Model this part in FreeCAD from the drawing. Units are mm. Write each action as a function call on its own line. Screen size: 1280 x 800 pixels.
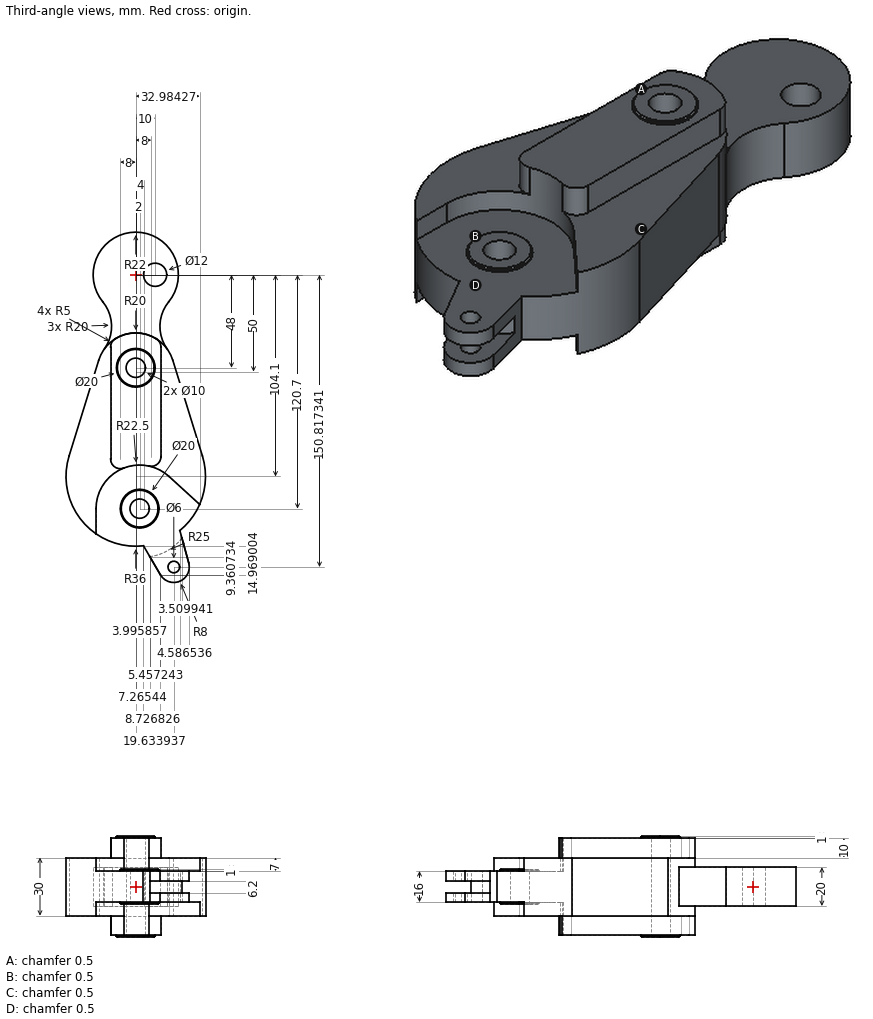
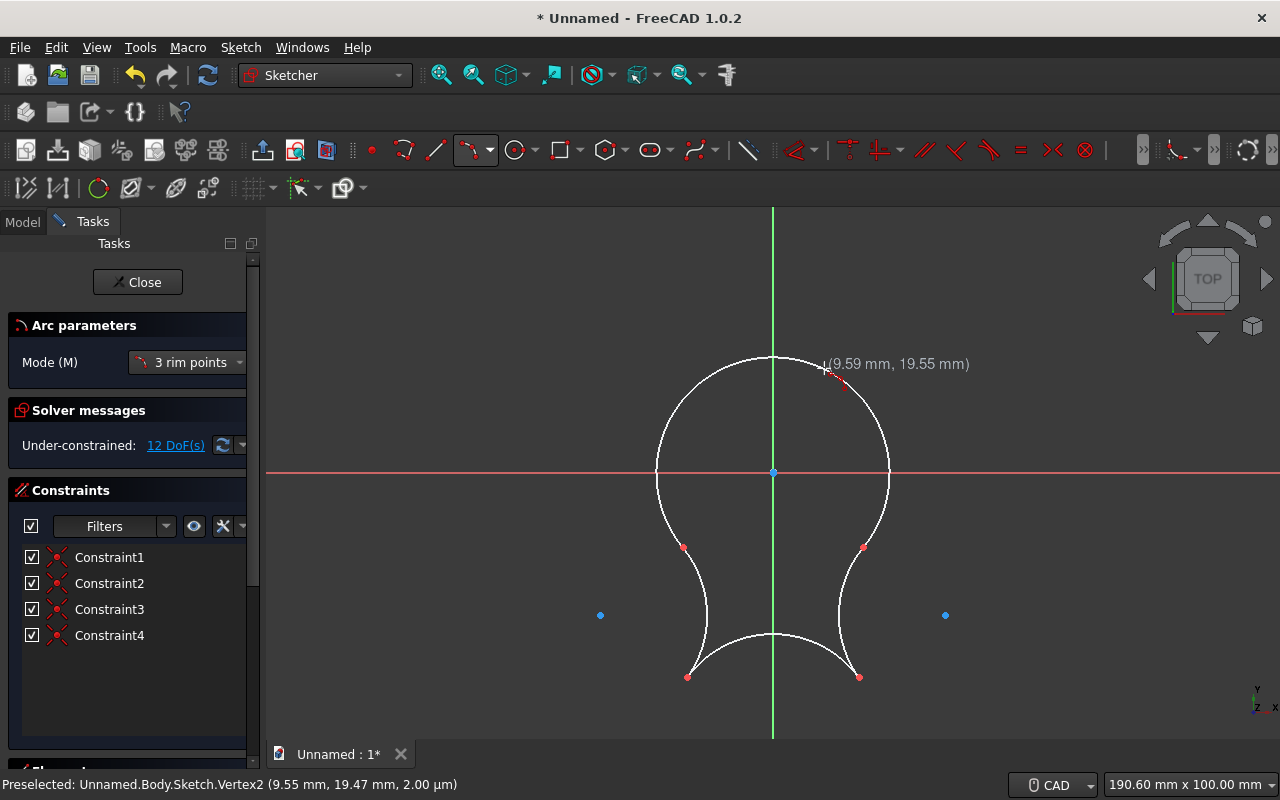
click(516, 150)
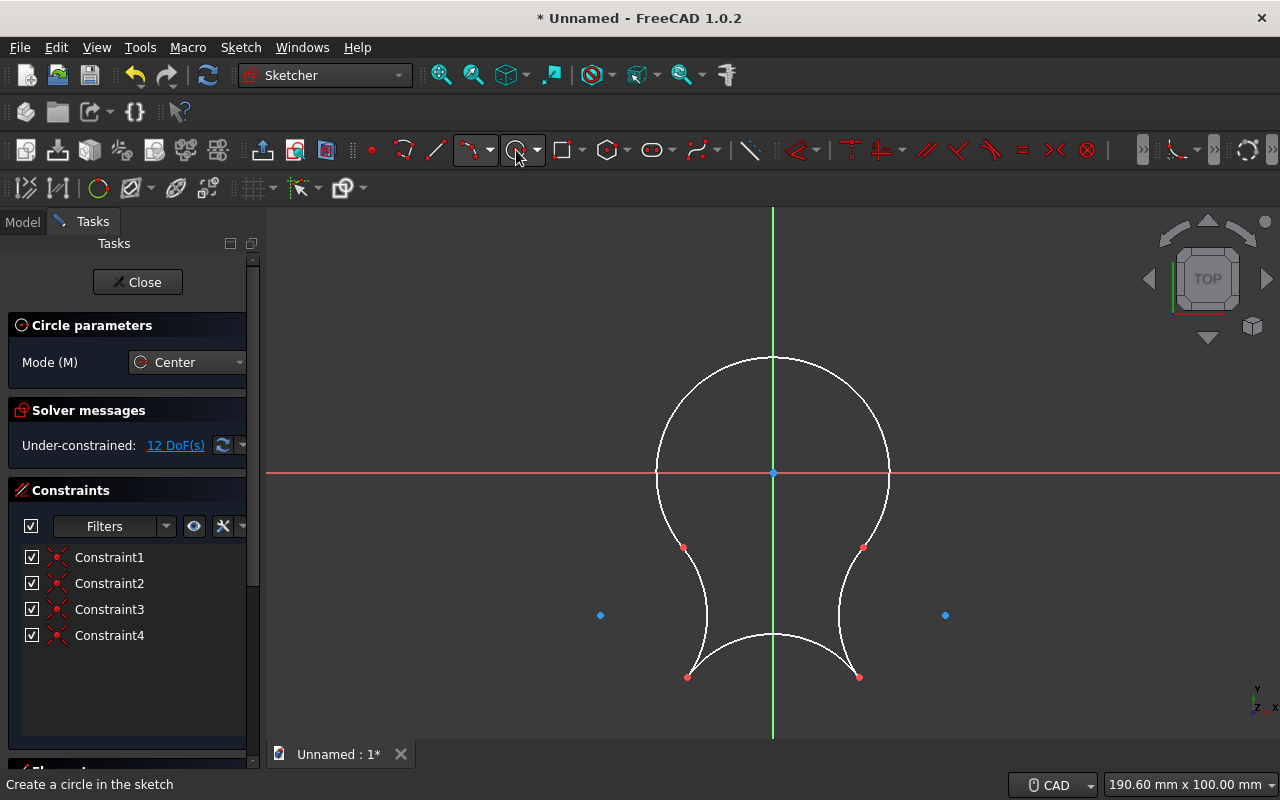
click(826, 473)
click(849, 450)
key(Escape)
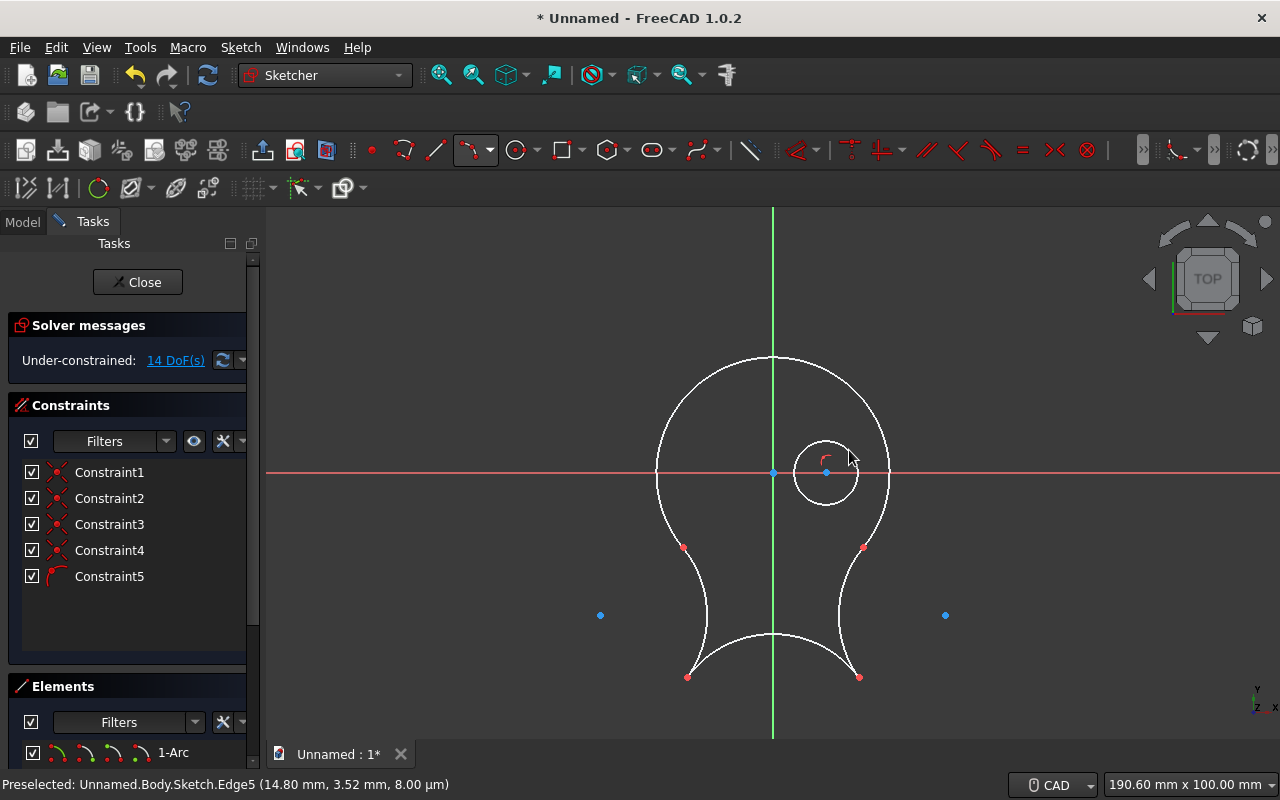
click(704, 640)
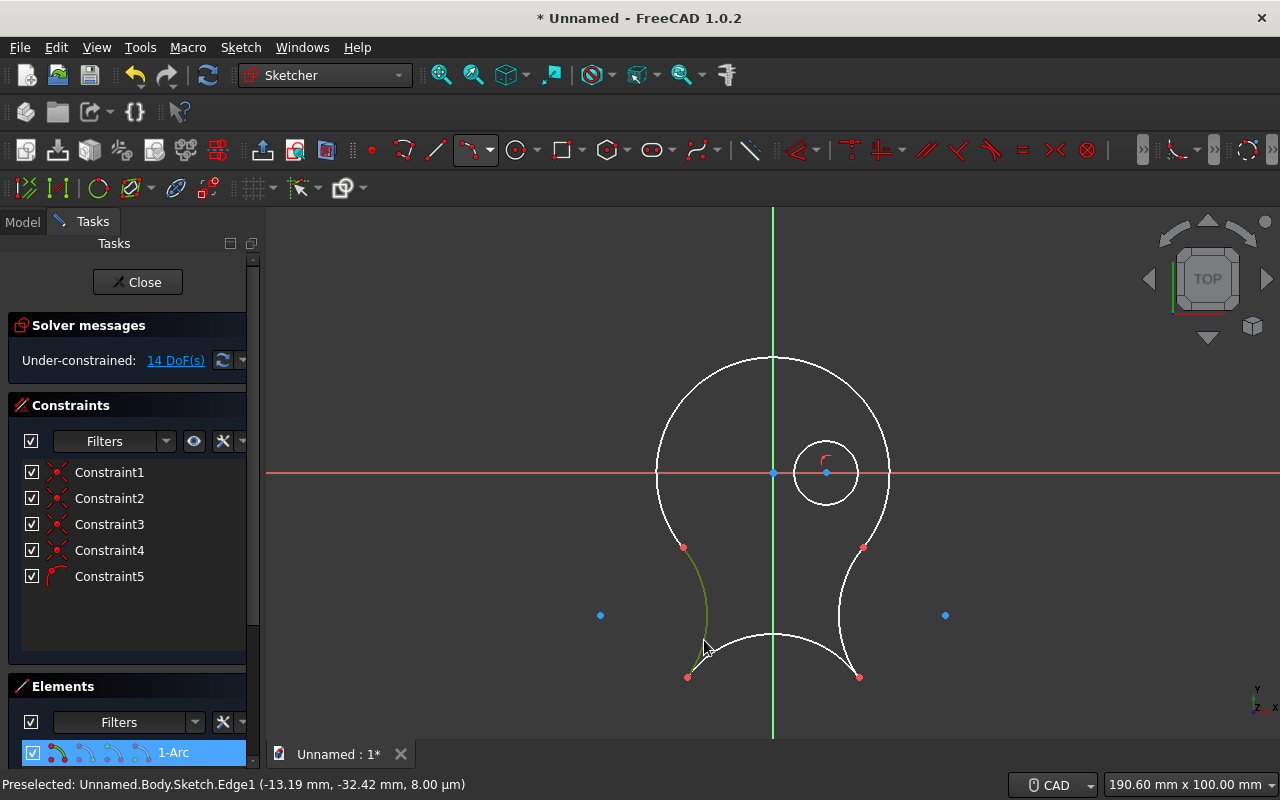
click(812, 642)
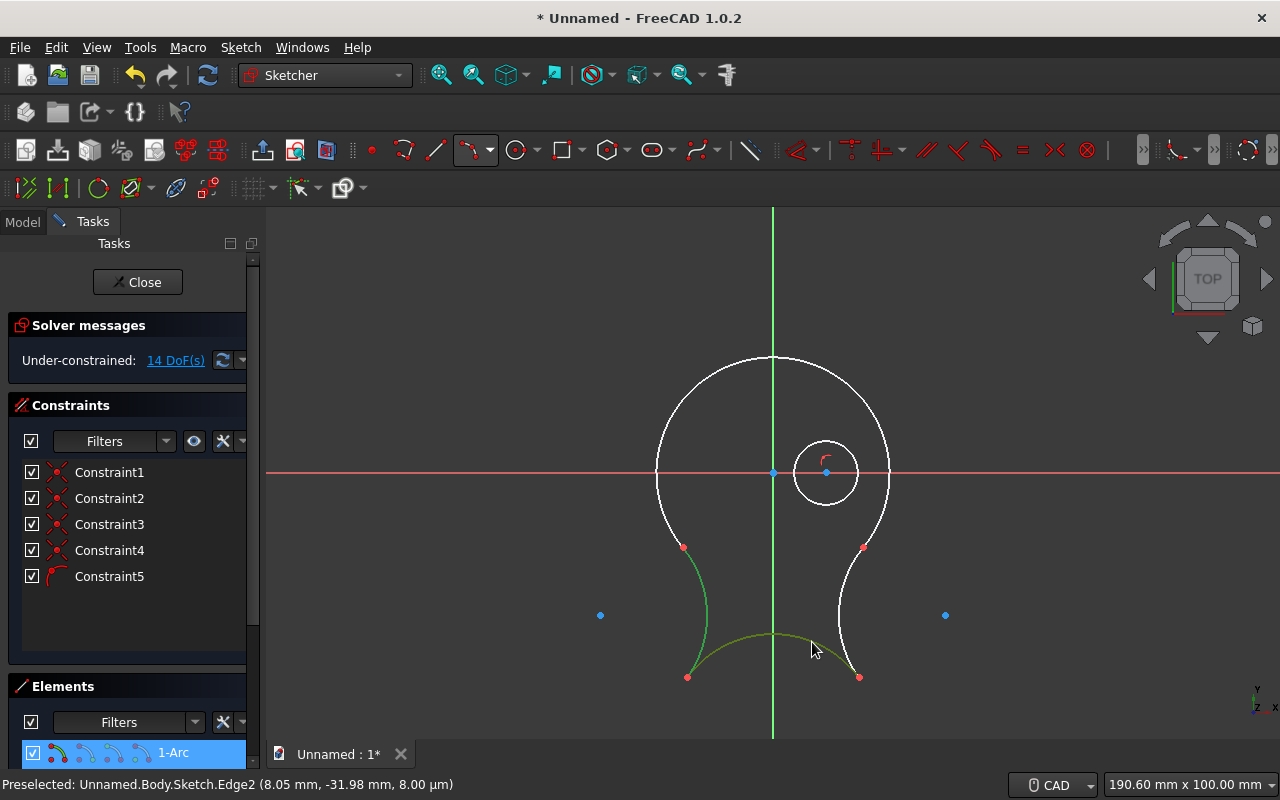
click(992, 150)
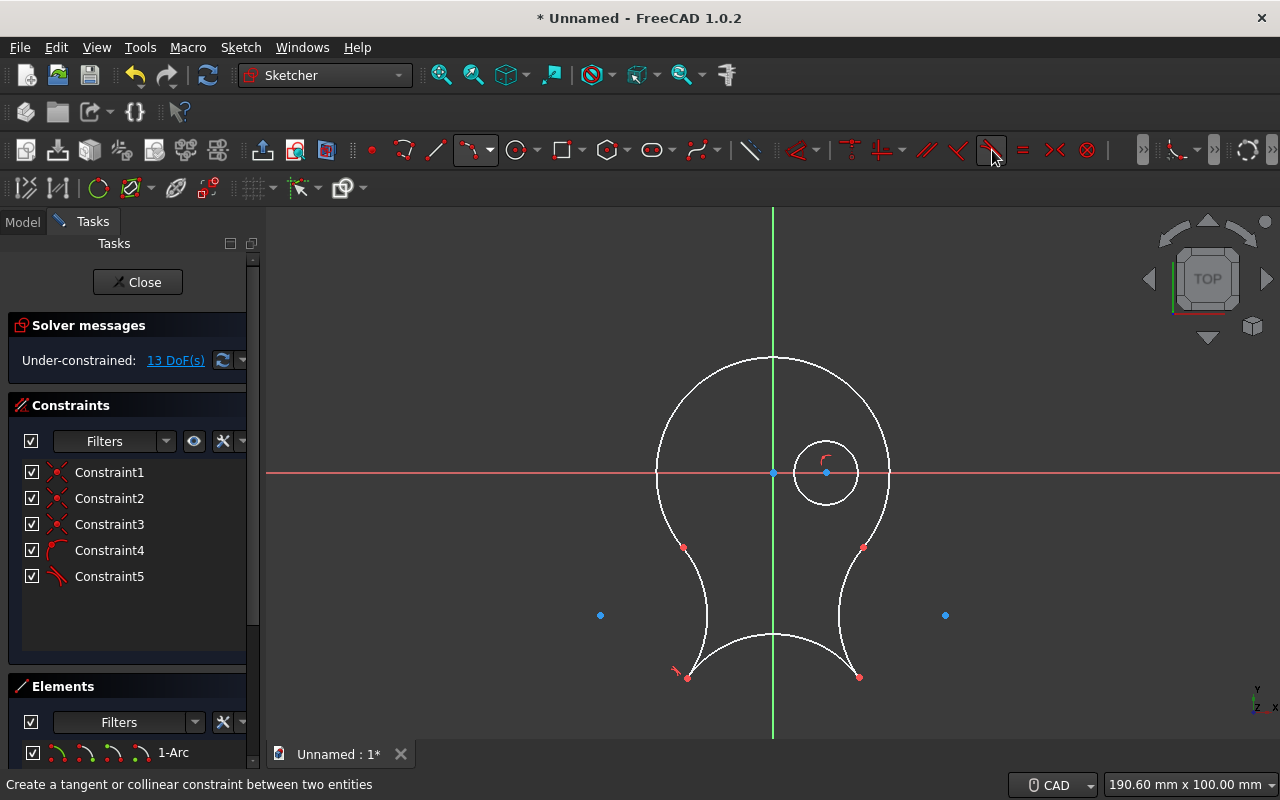
click(704, 640)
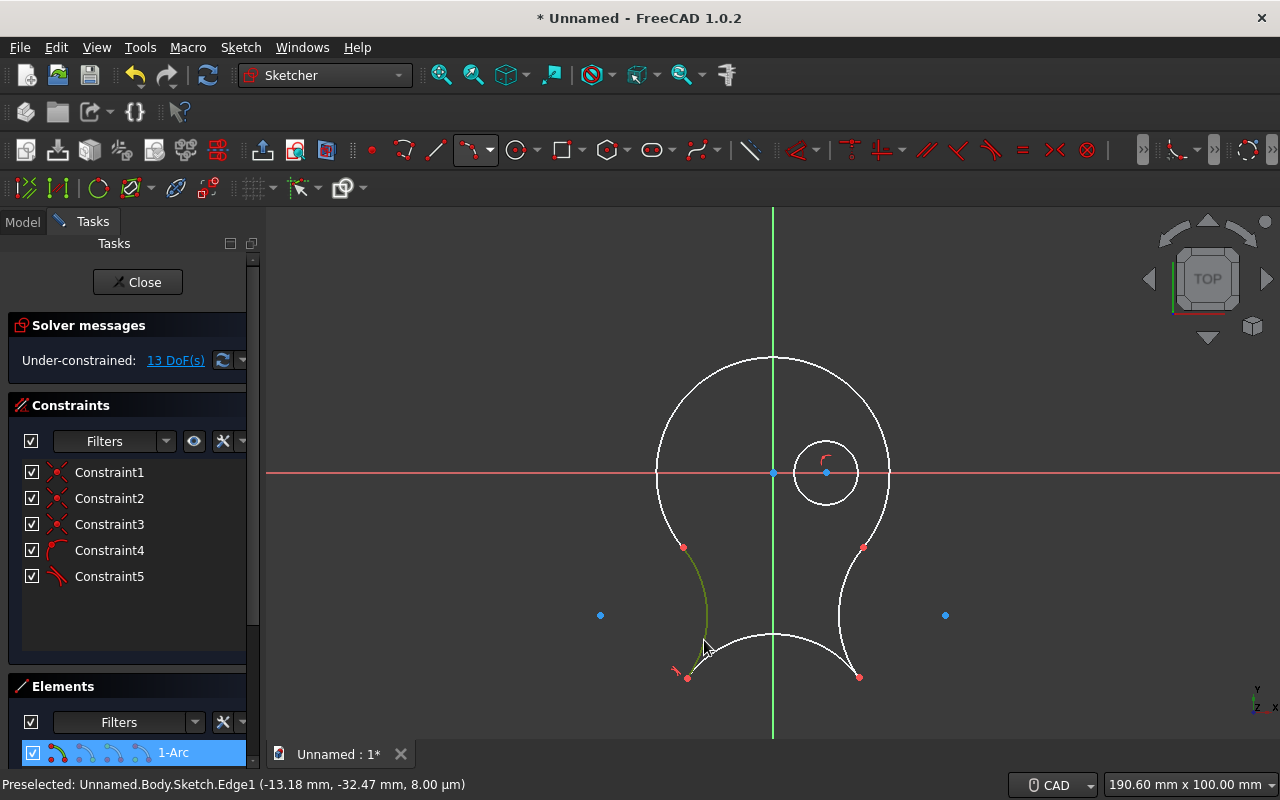
click(865, 402)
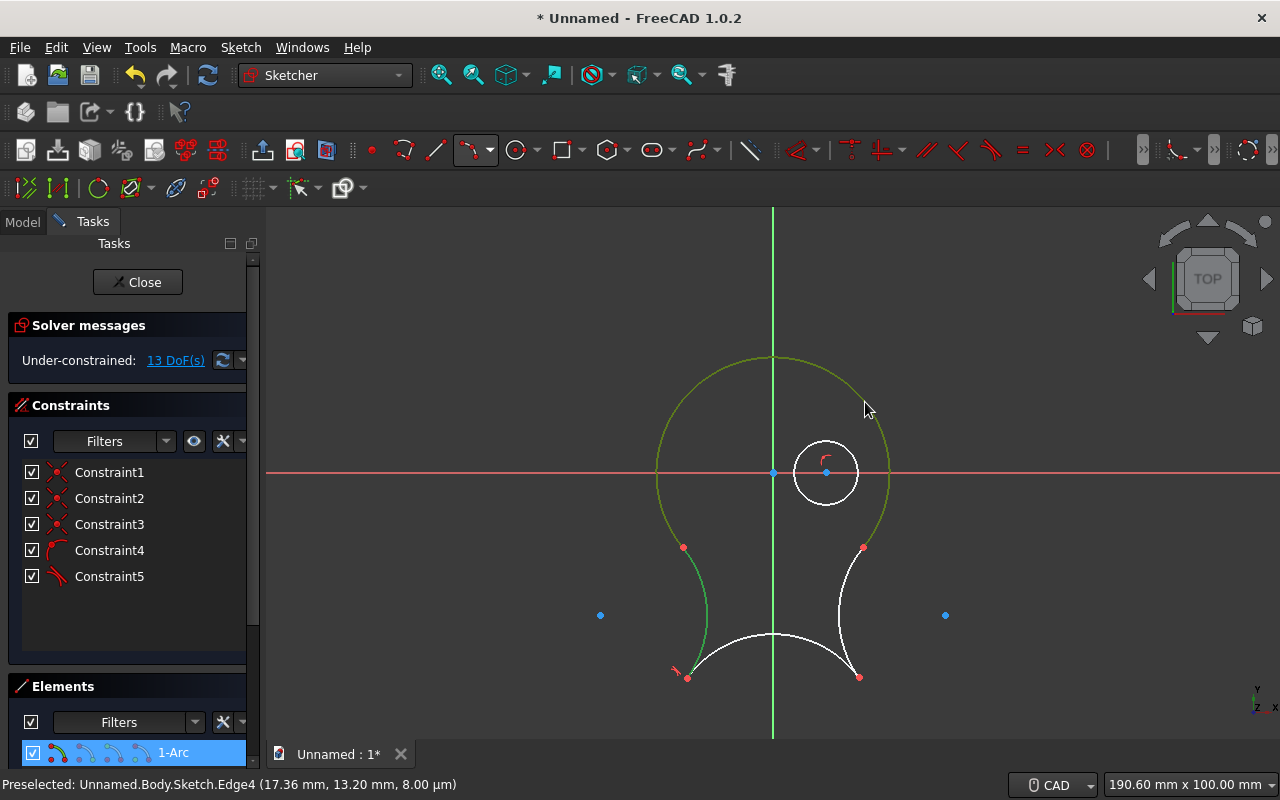
click(992, 150)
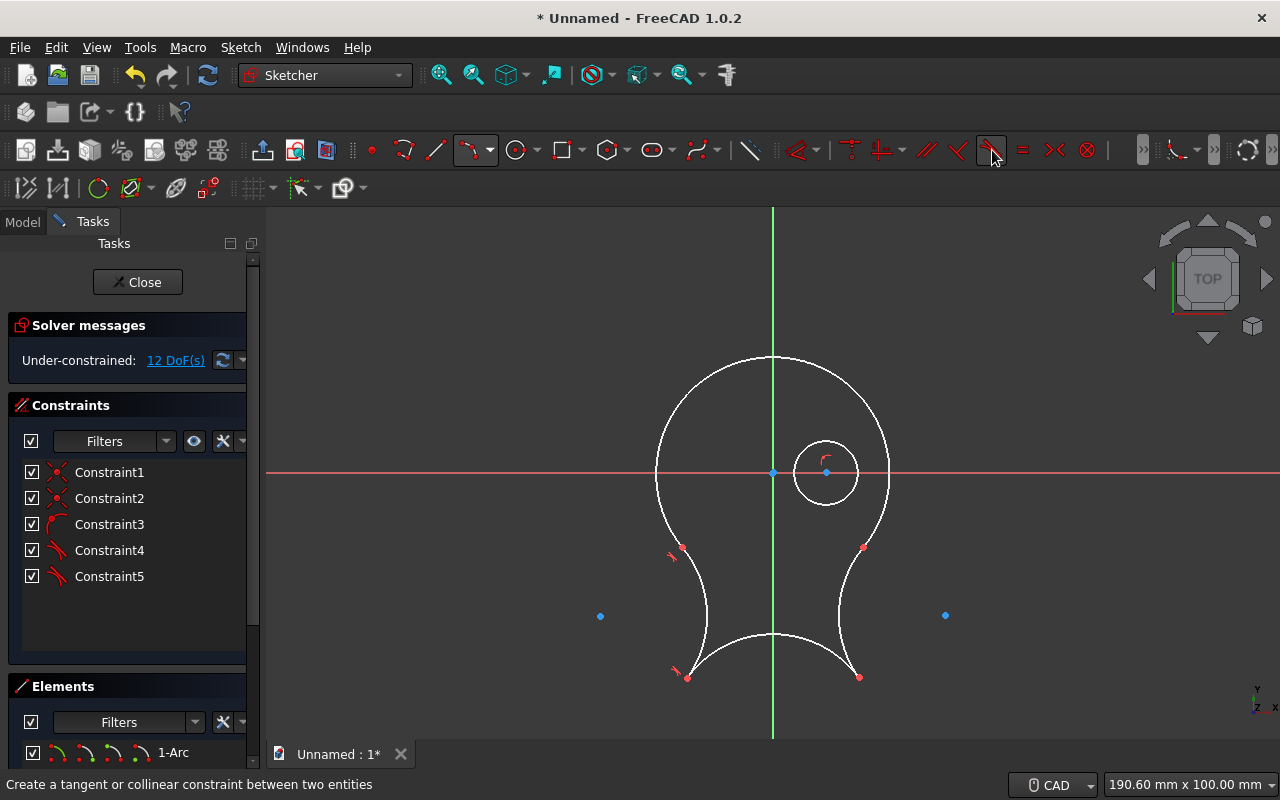
click(812, 642)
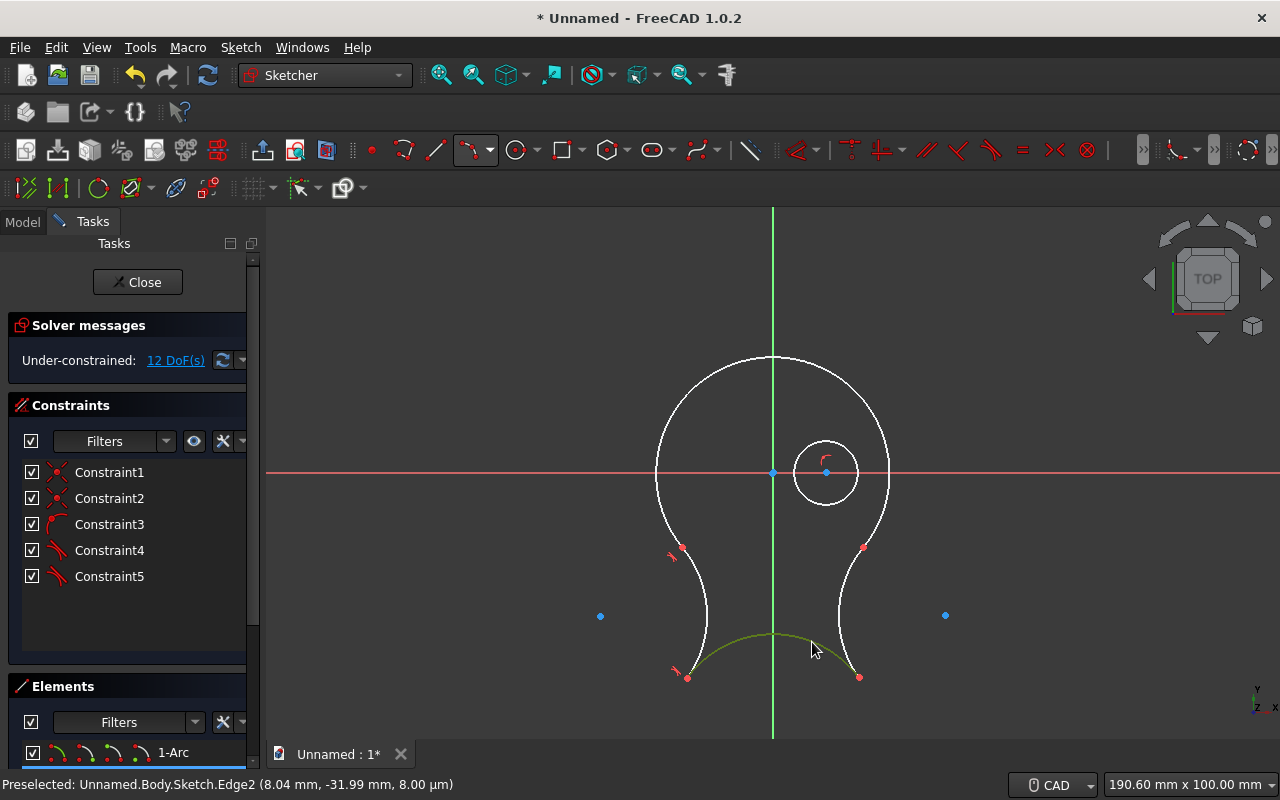
click(843, 585)